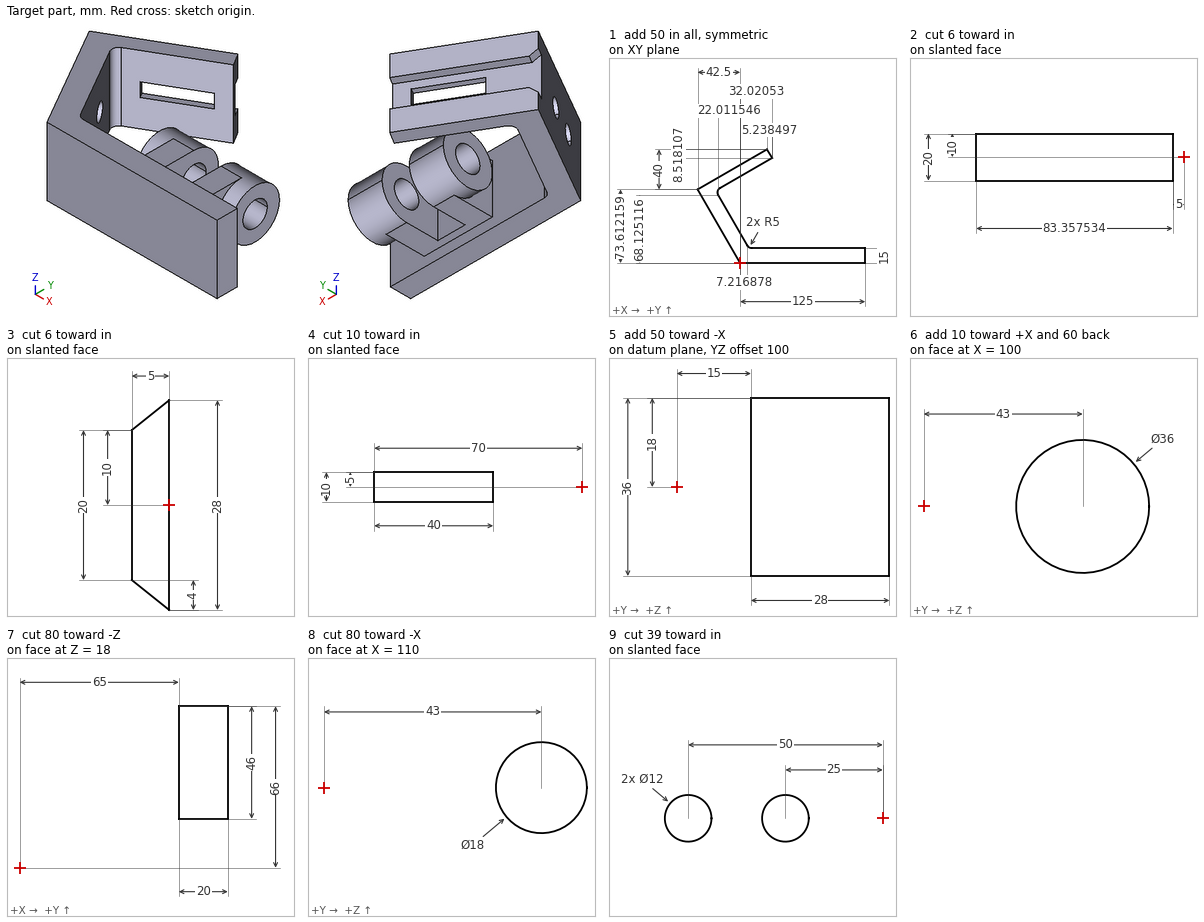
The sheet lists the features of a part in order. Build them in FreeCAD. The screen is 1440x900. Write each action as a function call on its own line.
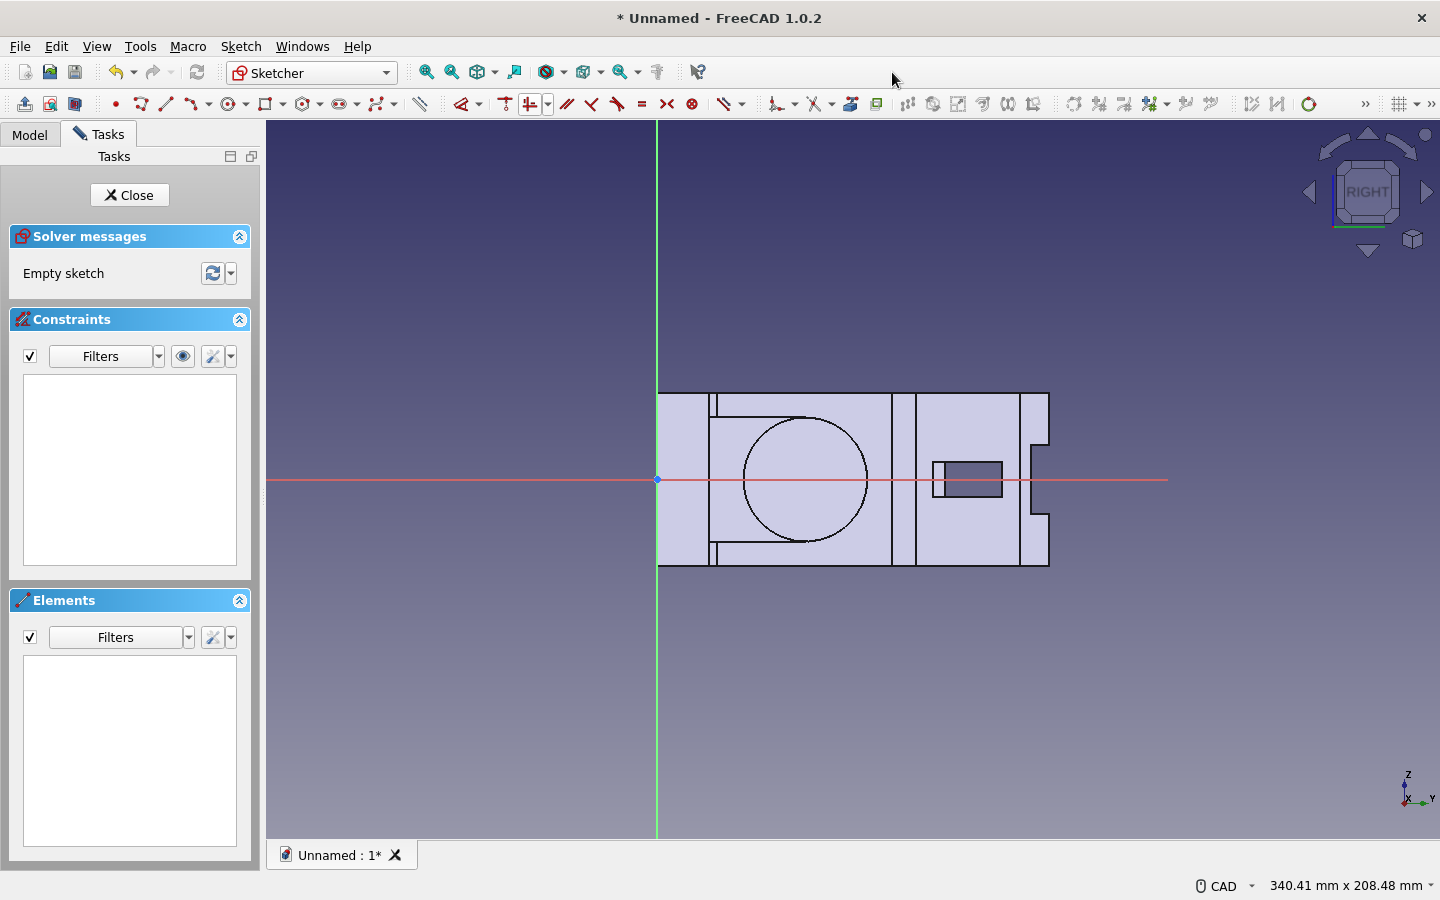
scroll(809, 480, up, 10)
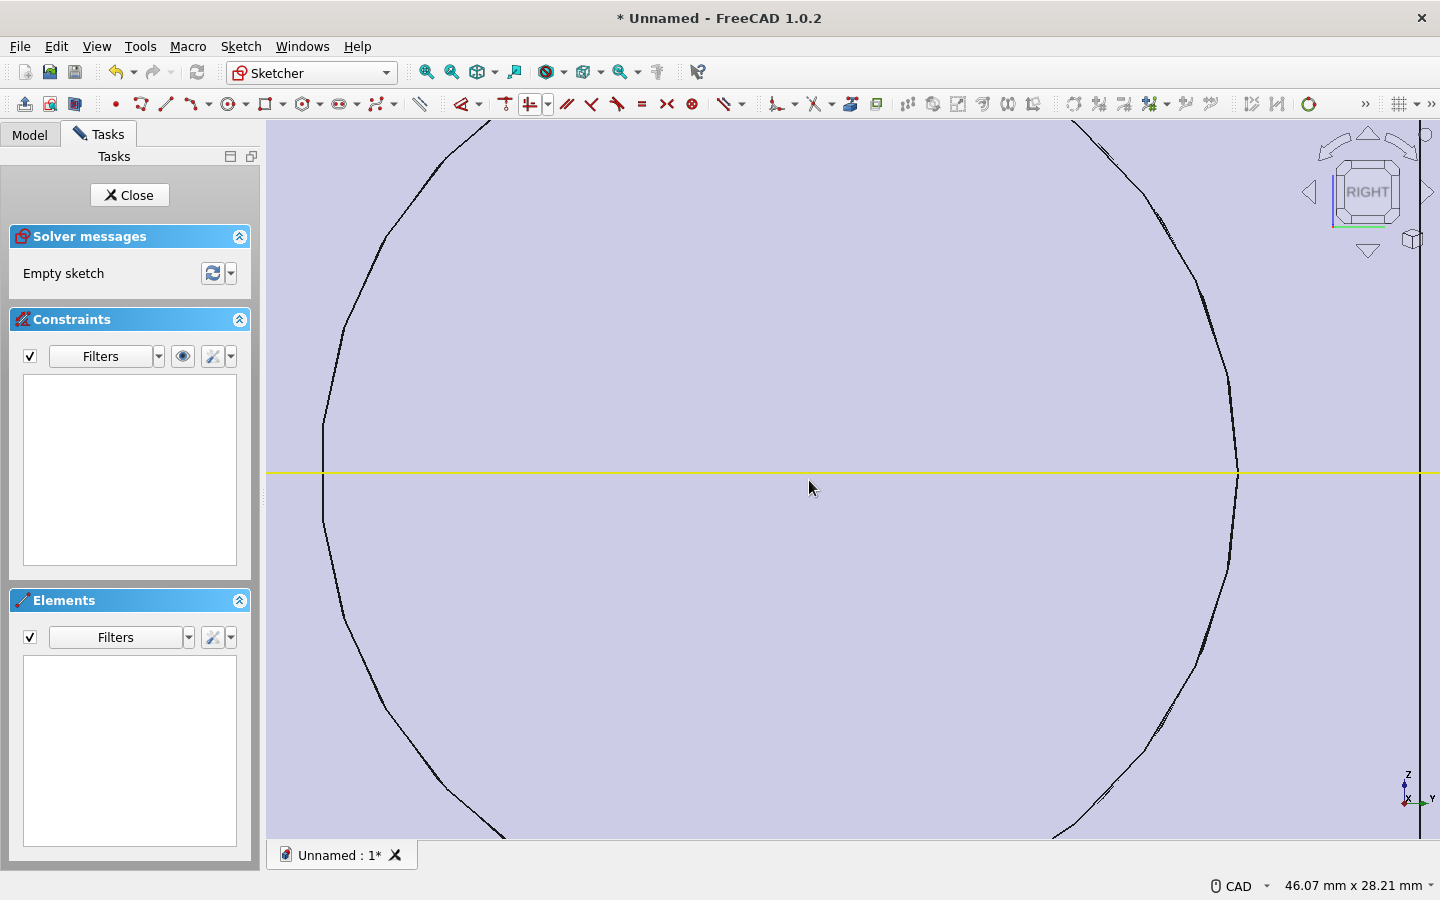
key(g)
key(c)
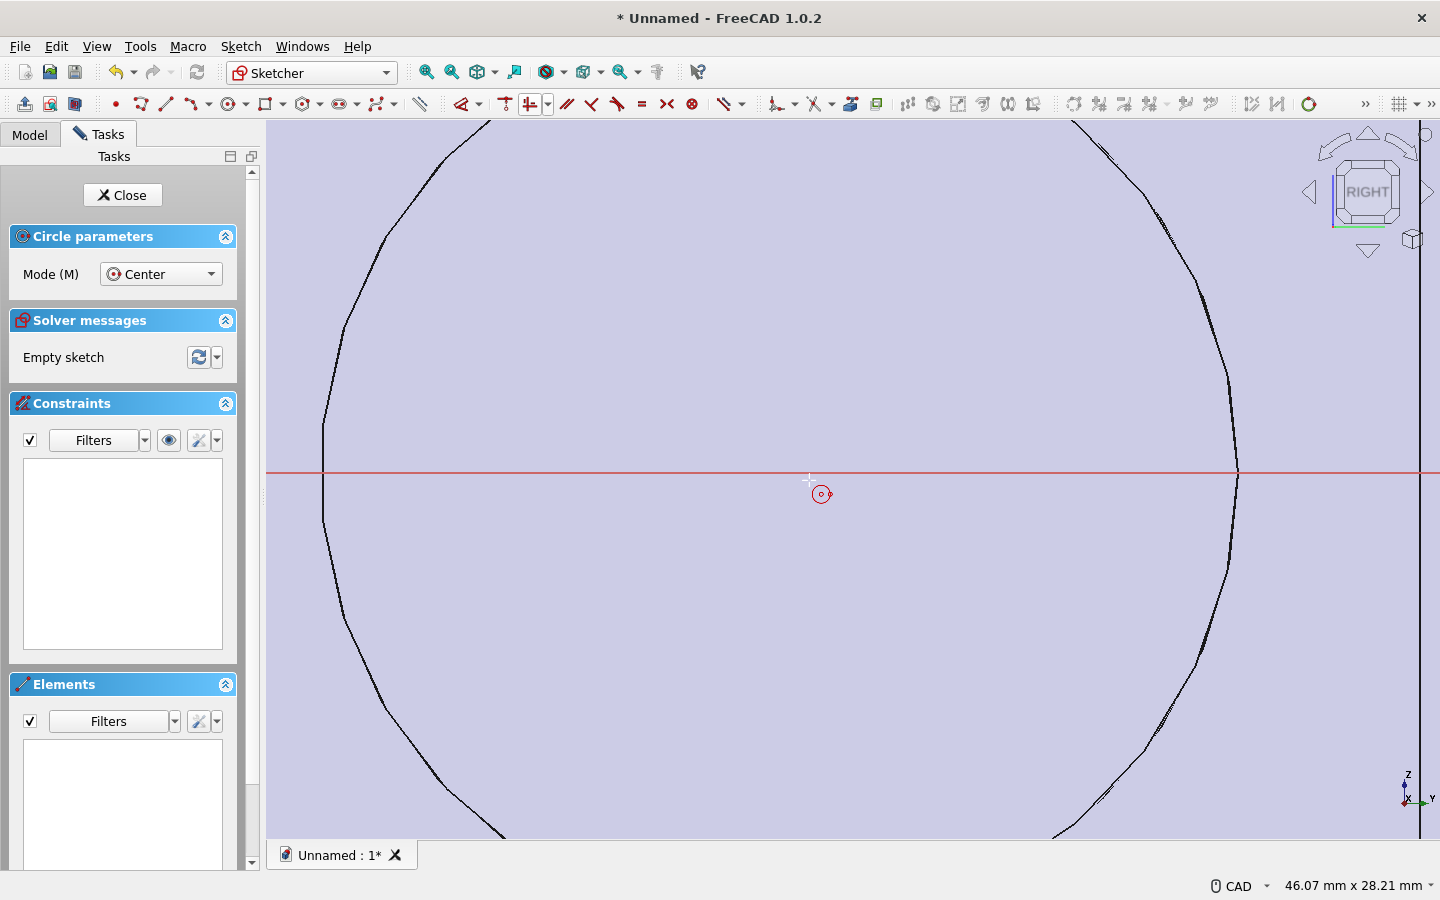
click(779, 473)
click(942, 311)
key(Escape)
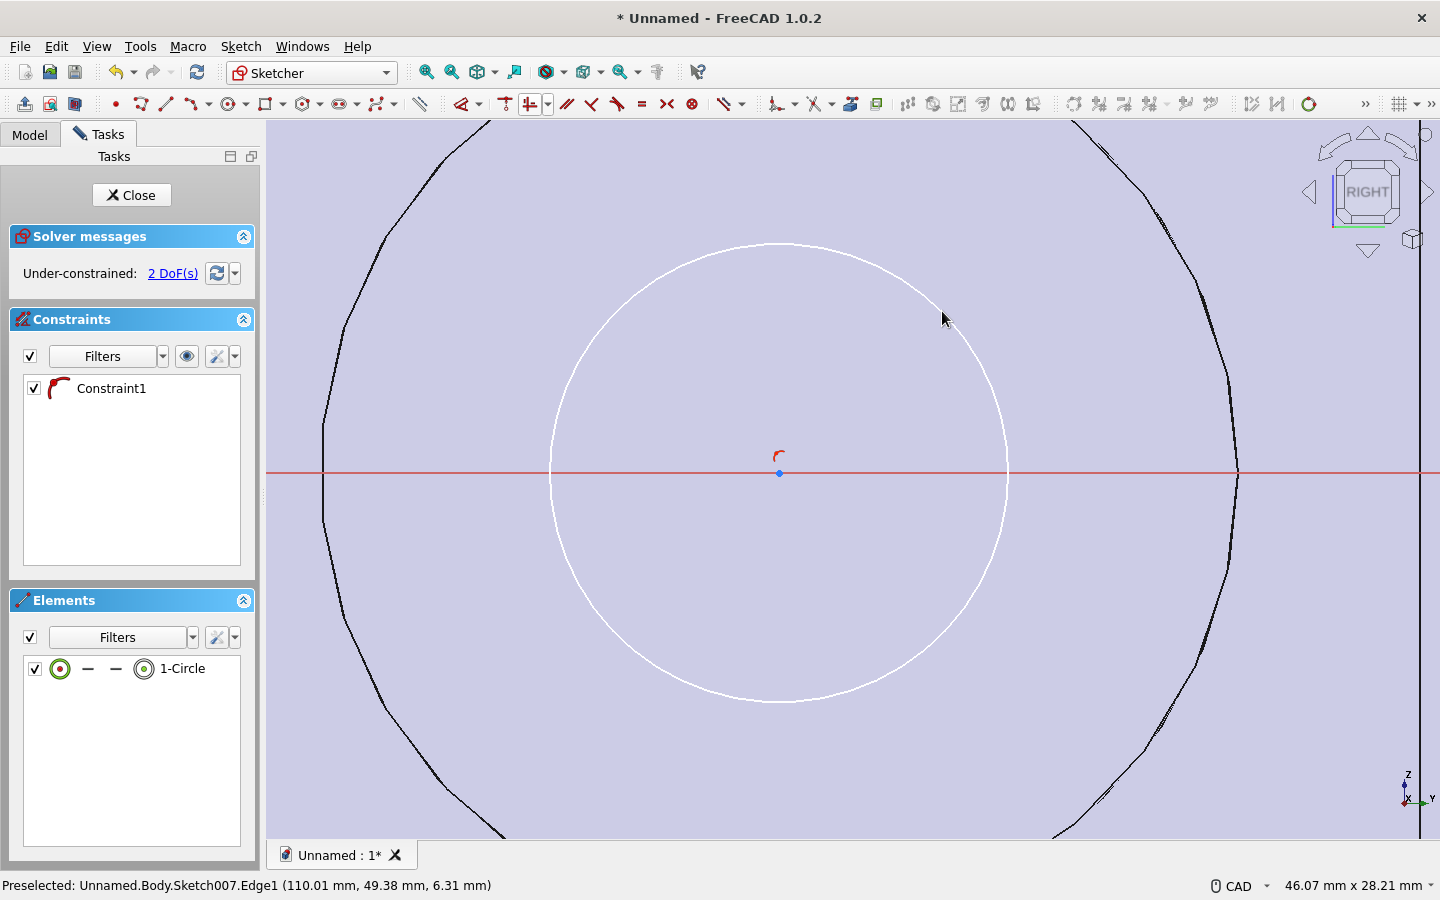
click(460, 104)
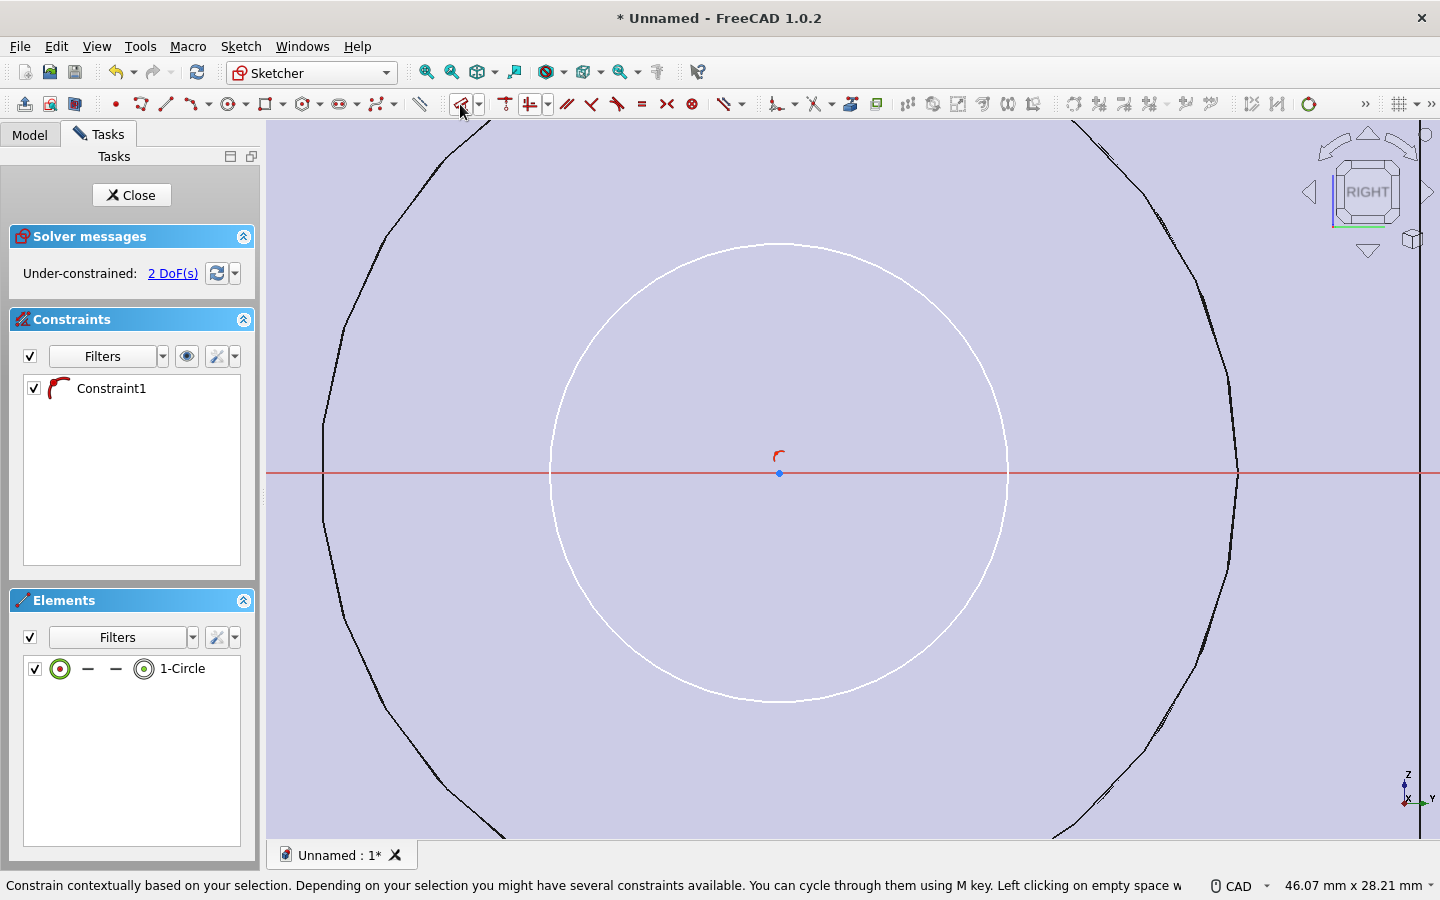
click(941, 311)
click(964, 288)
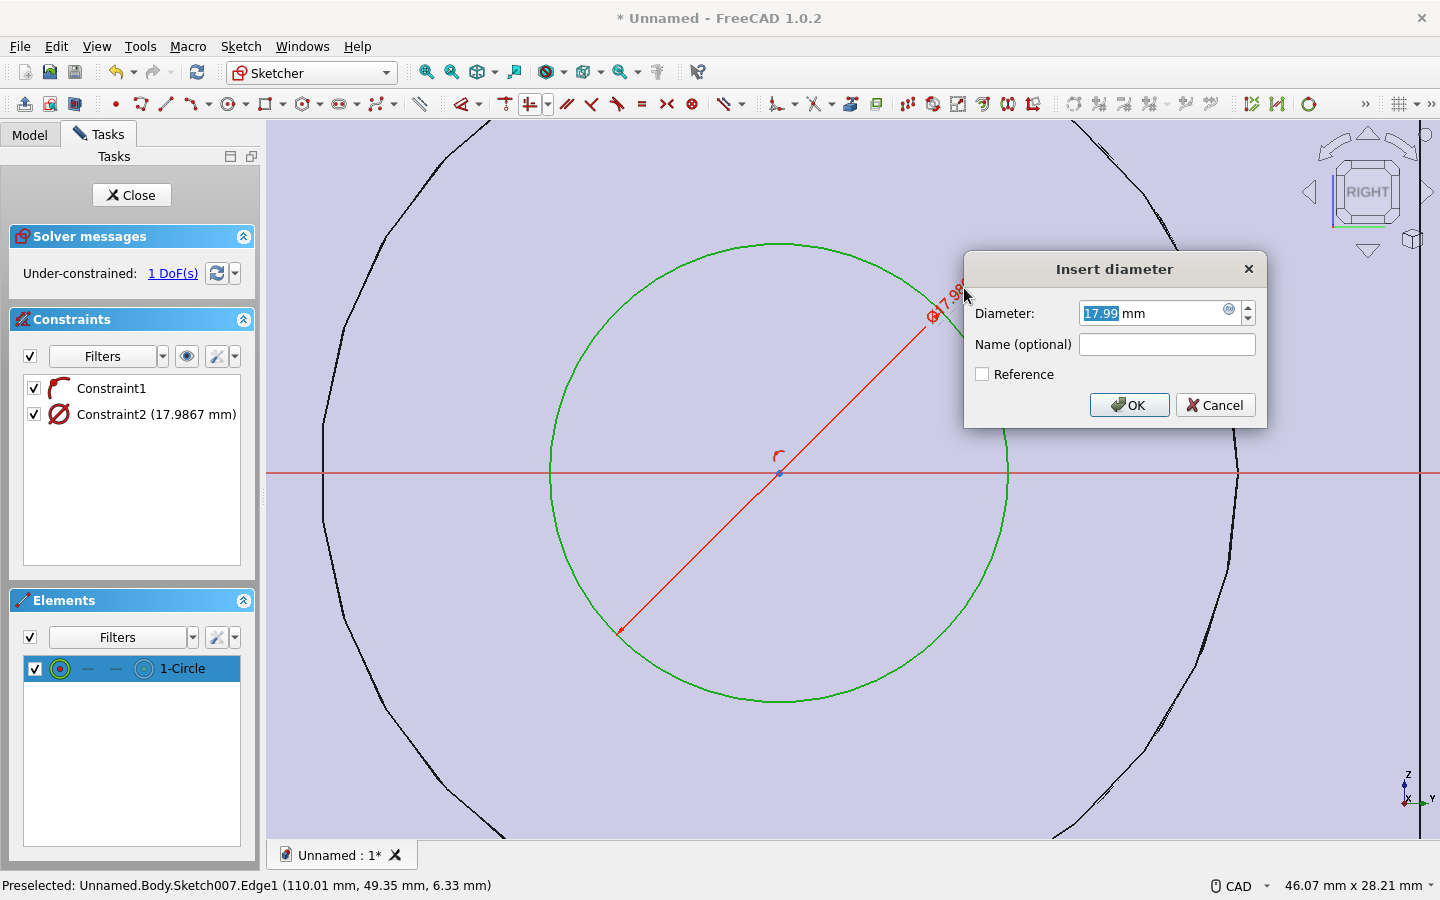
text(18)
key(Return)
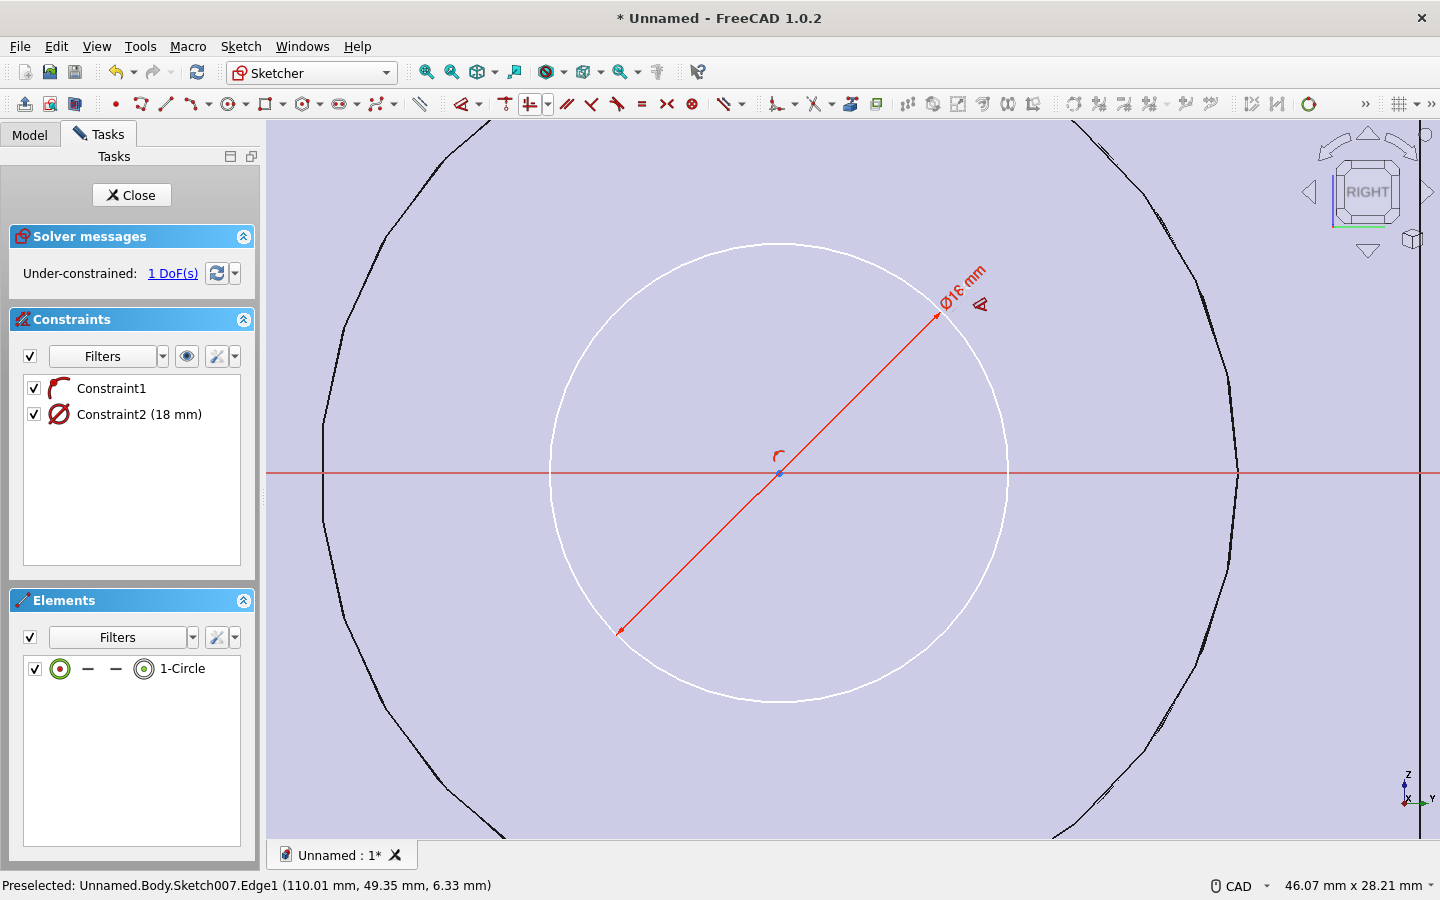
click(779, 473)
click(536, 507)